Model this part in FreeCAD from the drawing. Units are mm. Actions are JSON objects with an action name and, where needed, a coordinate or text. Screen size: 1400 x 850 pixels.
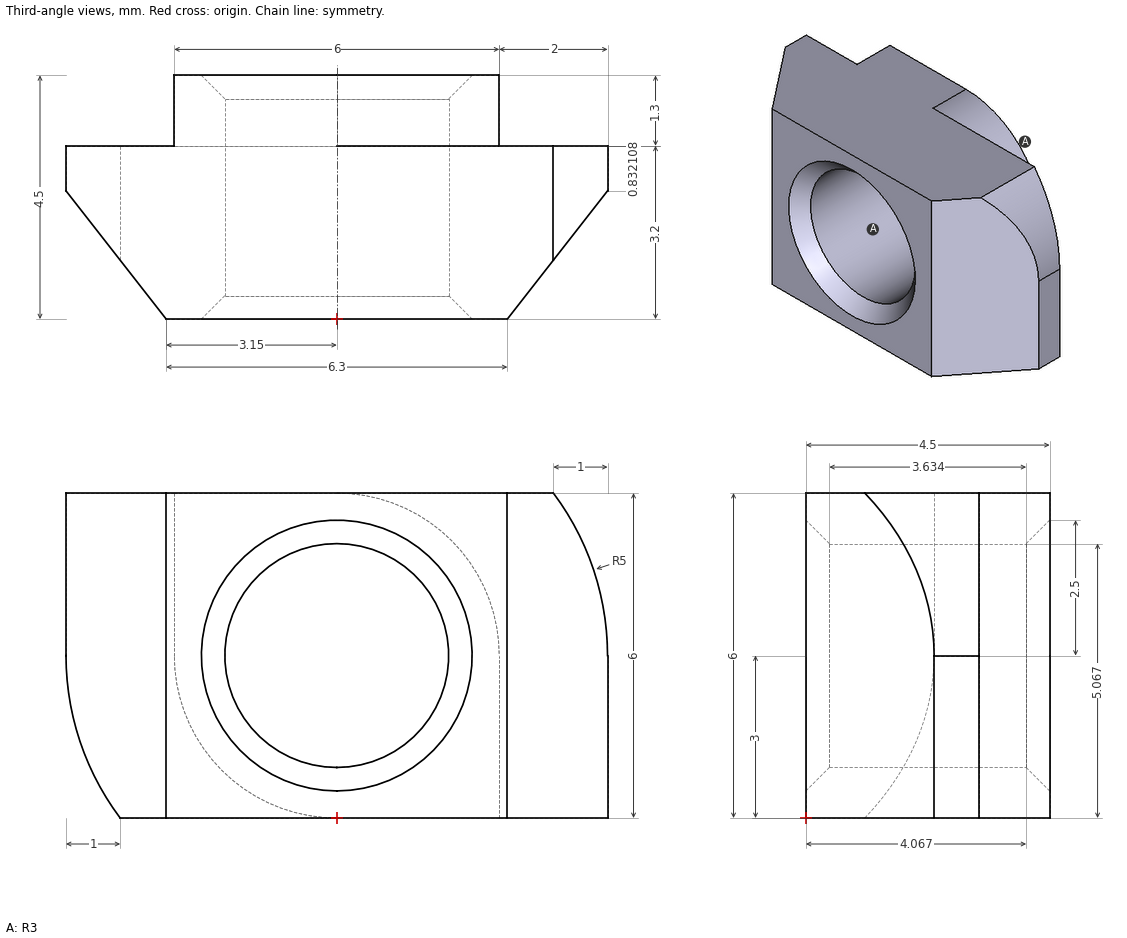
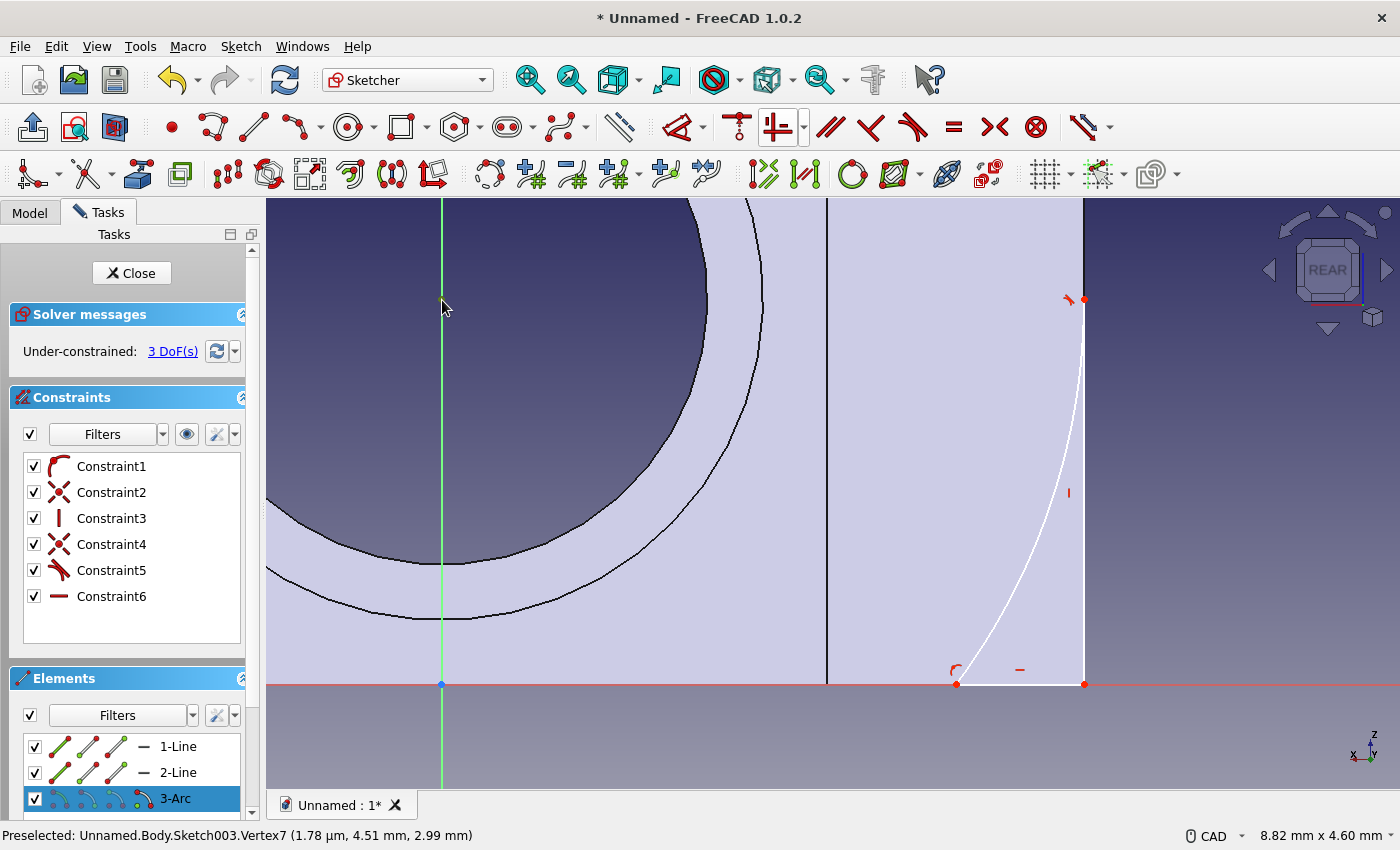
{"action": "left_click", "coordinate": [442, 723]}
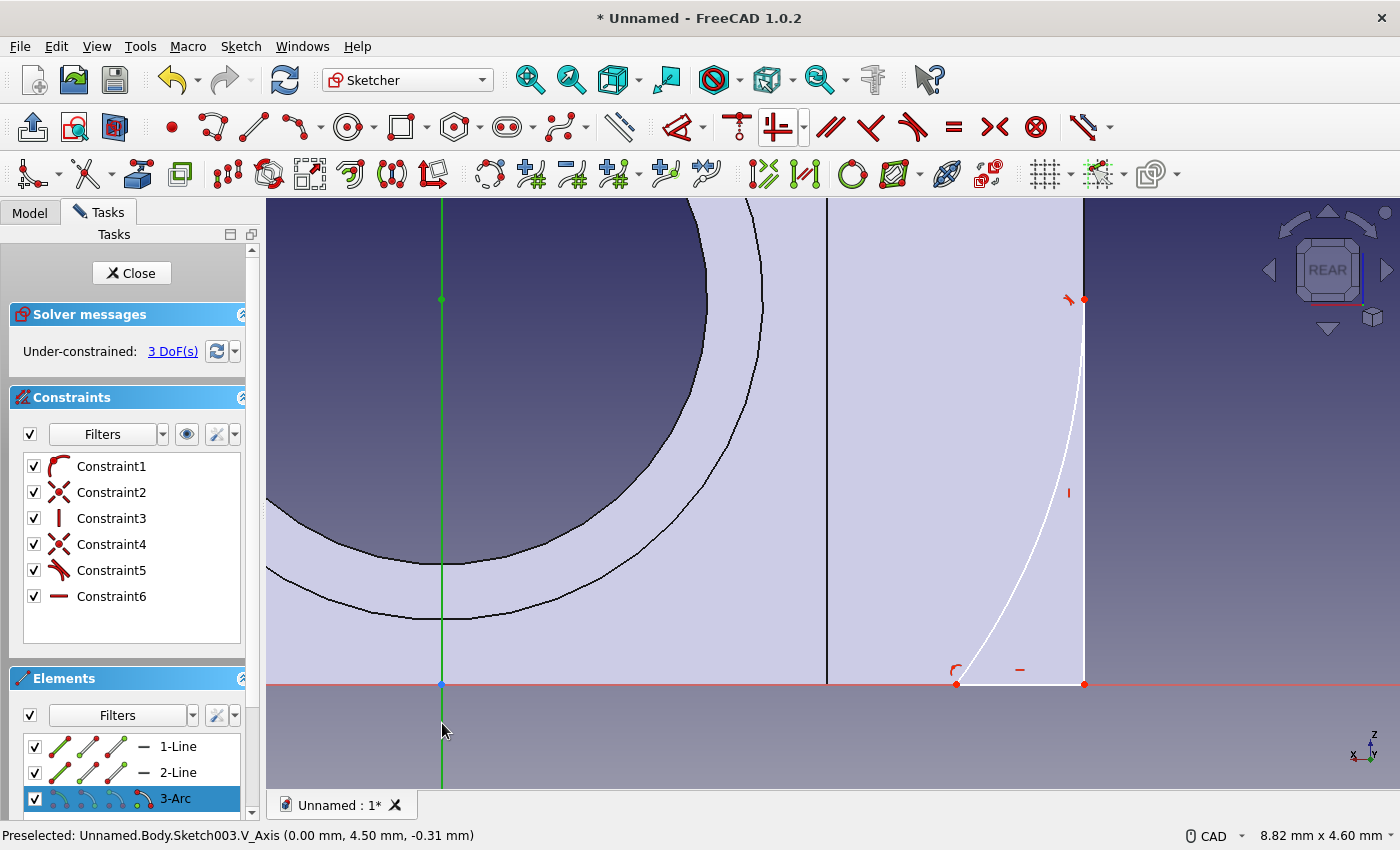
{"action": "left_click", "coordinate": [737, 128]}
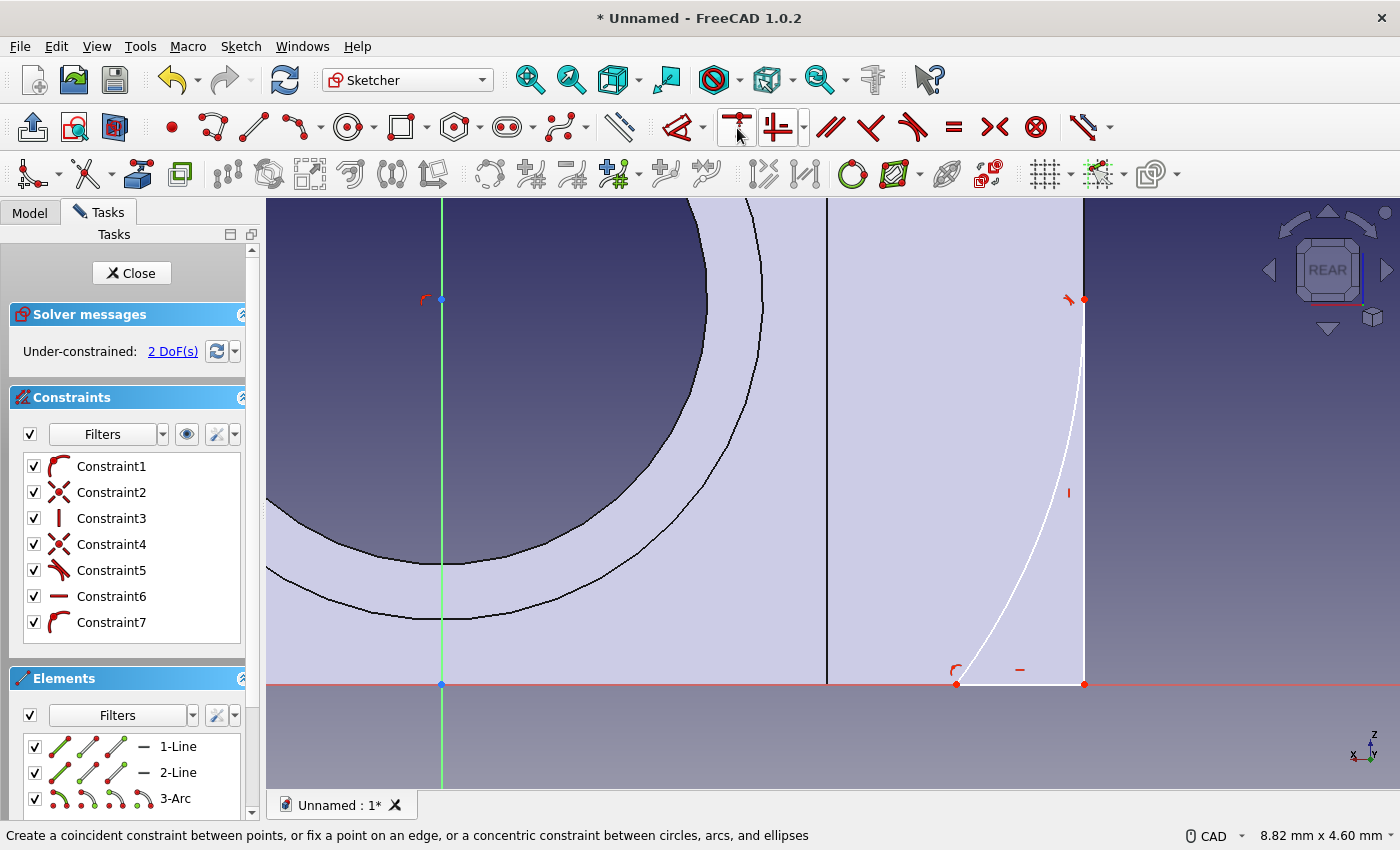
{"action": "left_click", "coordinate": [676, 128]}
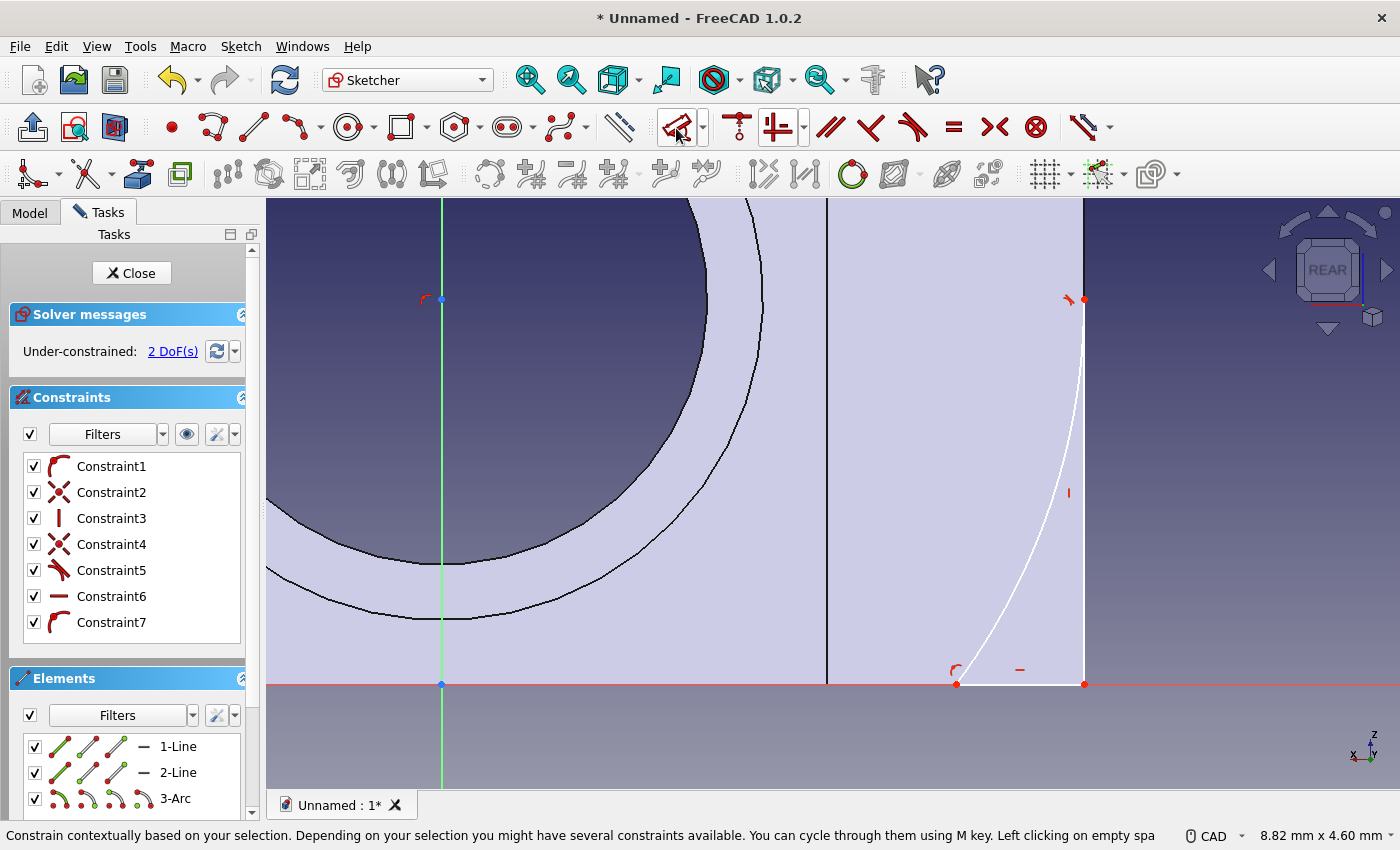
{"action": "left_click", "coordinate": [1020, 579]}
{"action": "left_click", "coordinate": [1049, 593]}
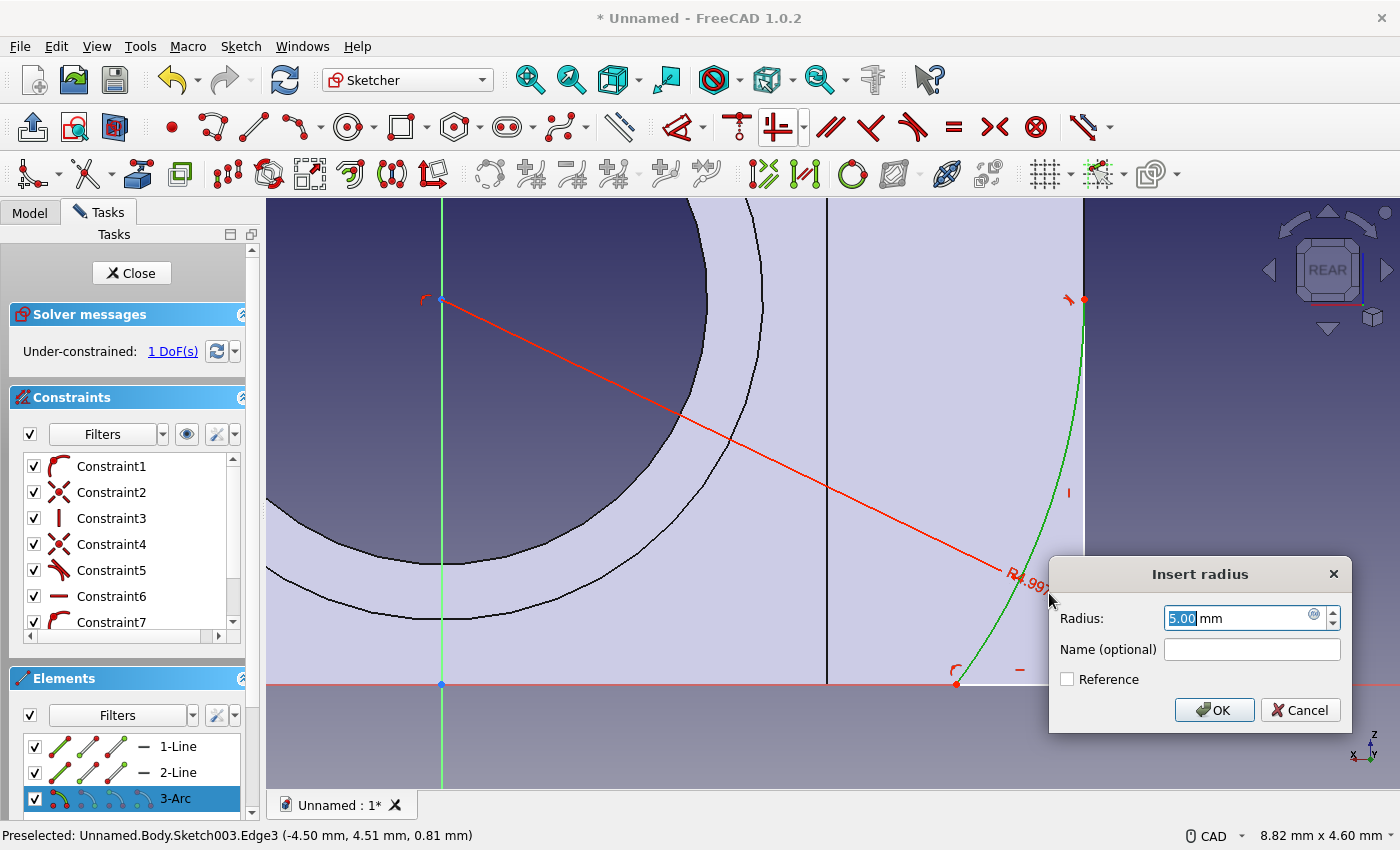
{"action": "type", "text": "5"}
{"action": "key", "text": "Return"}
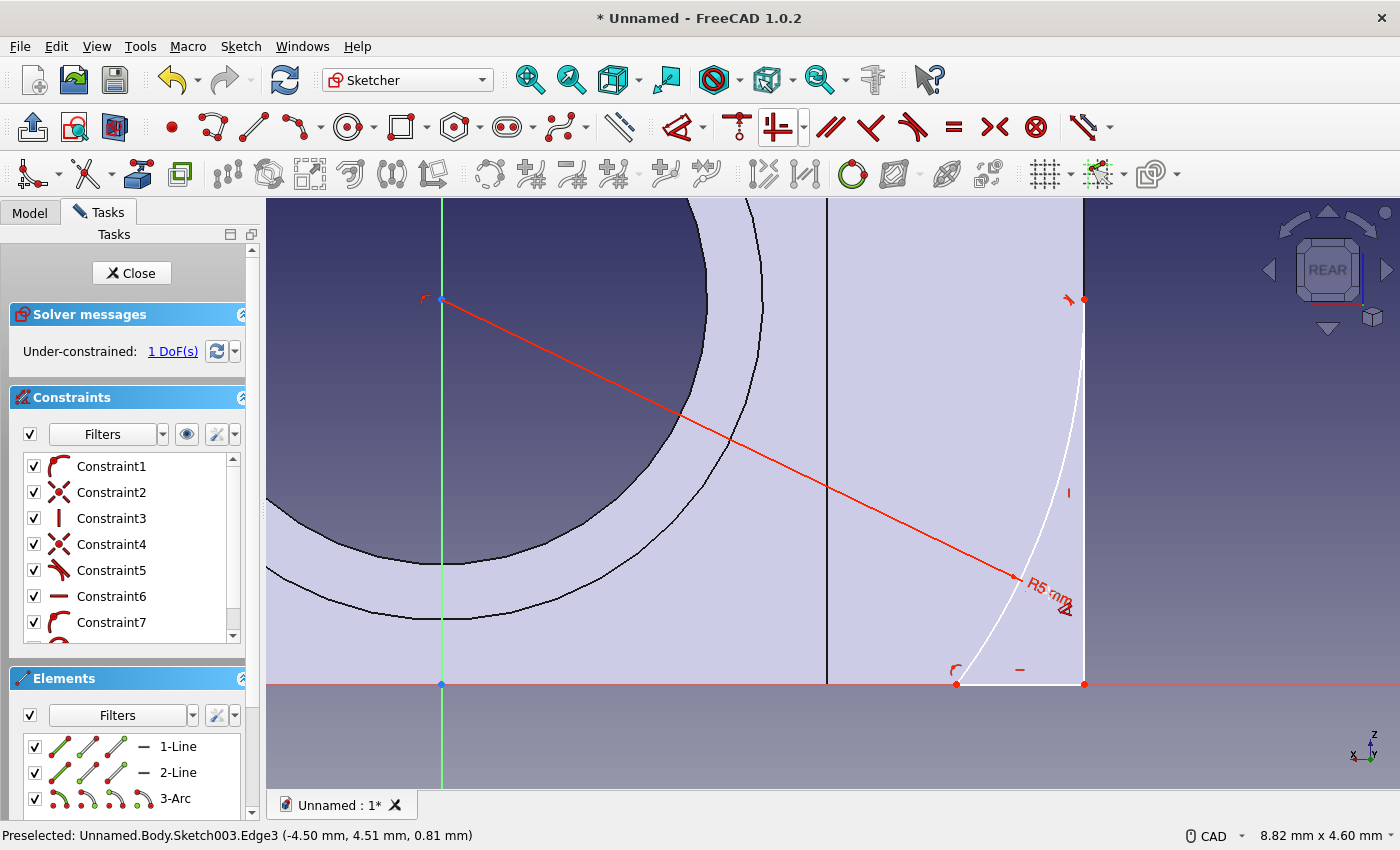
{"action": "left_click", "coordinate": [995, 685]}
{"action": "left_click", "coordinate": [1020, 719]}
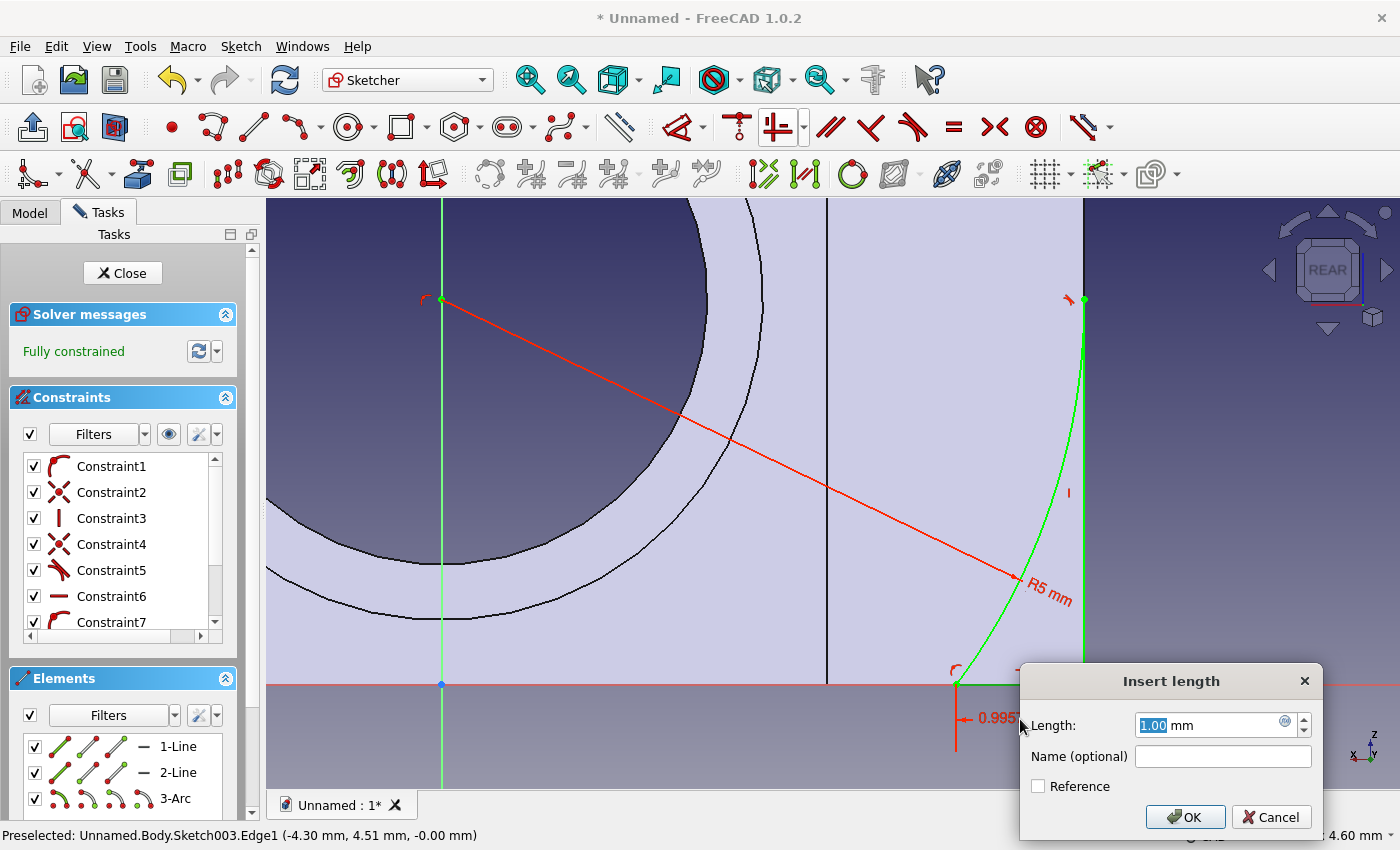
{"action": "type", "text": "1"}
{"action": "key", "text": "Return"}
{"action": "key", "text": "Escape"}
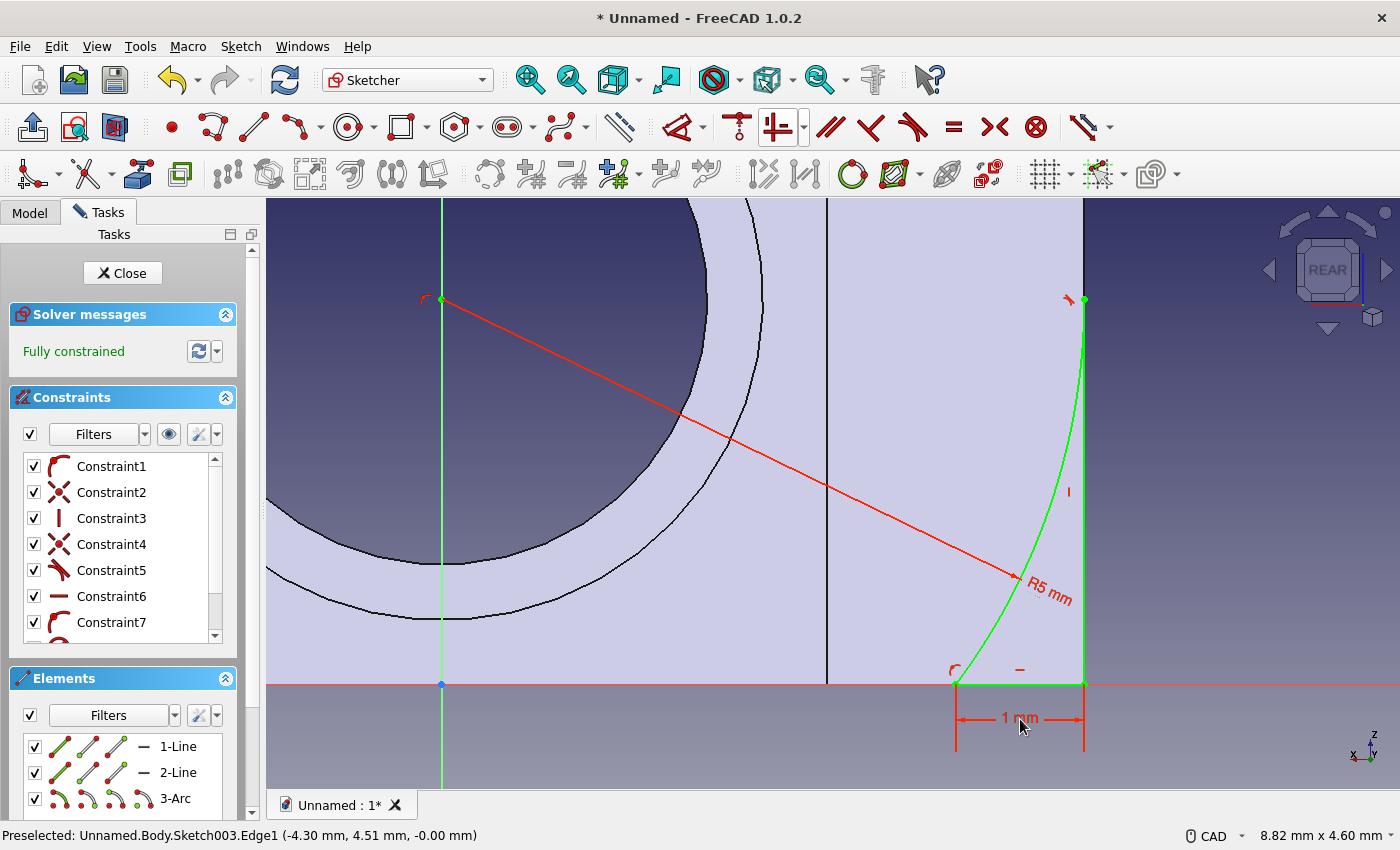
{"action": "left_click", "coordinate": [123, 273]}